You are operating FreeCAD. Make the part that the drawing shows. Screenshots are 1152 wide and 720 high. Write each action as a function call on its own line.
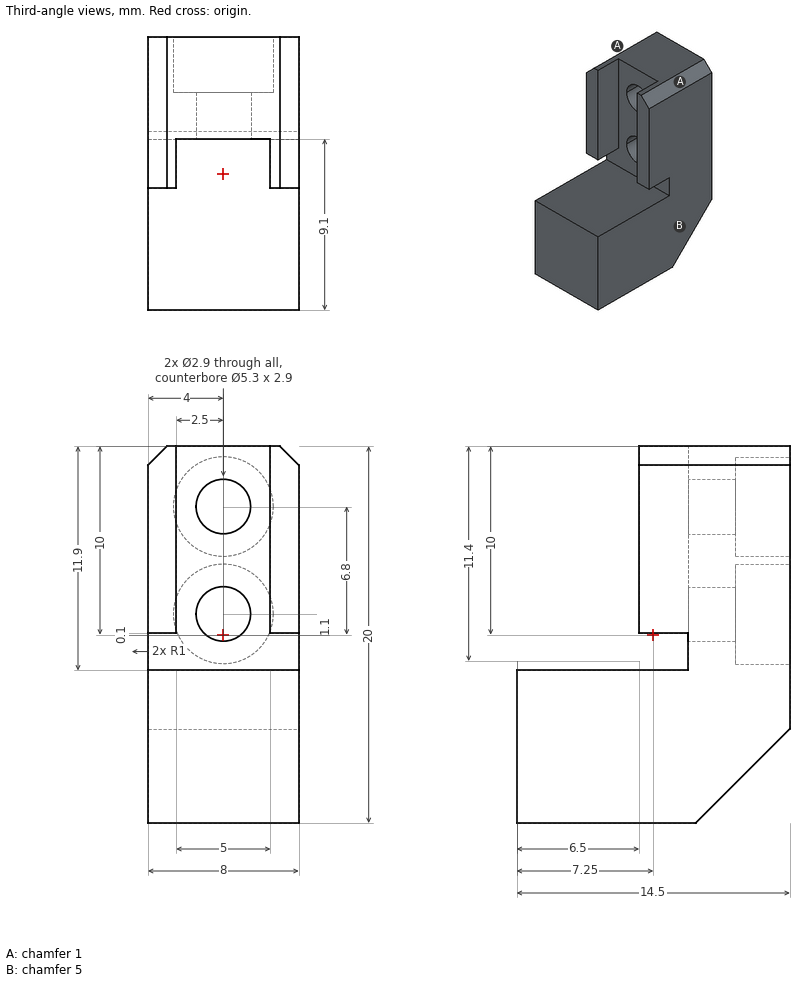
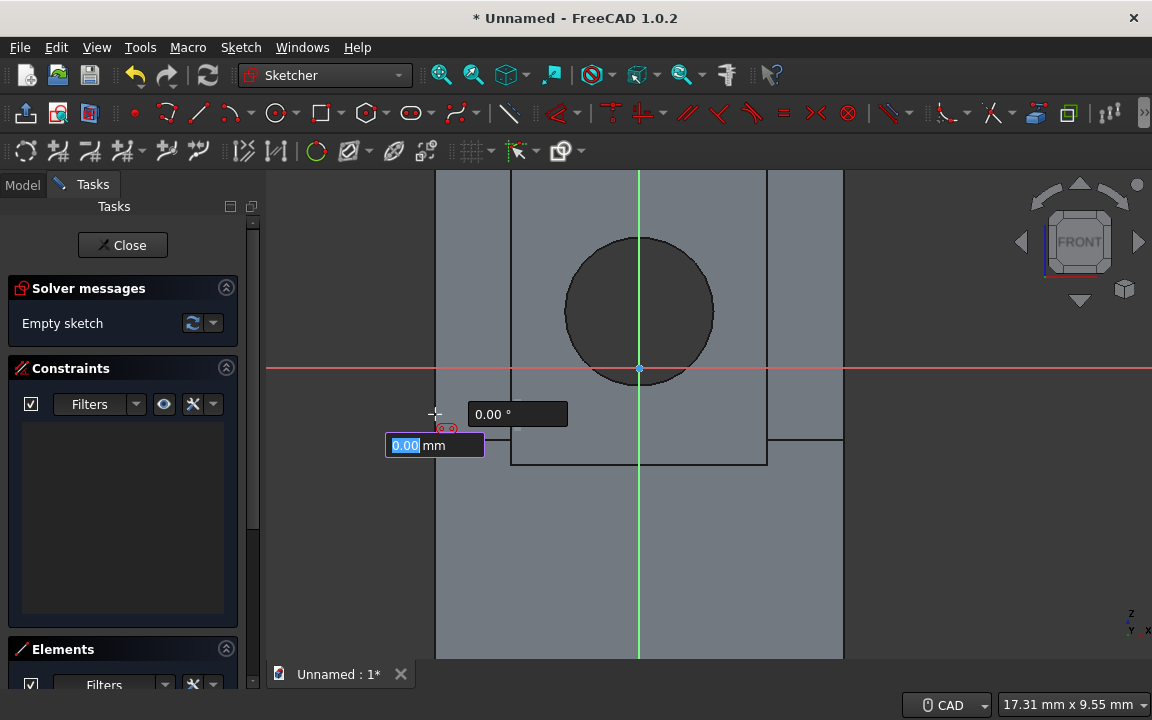
click(844, 414)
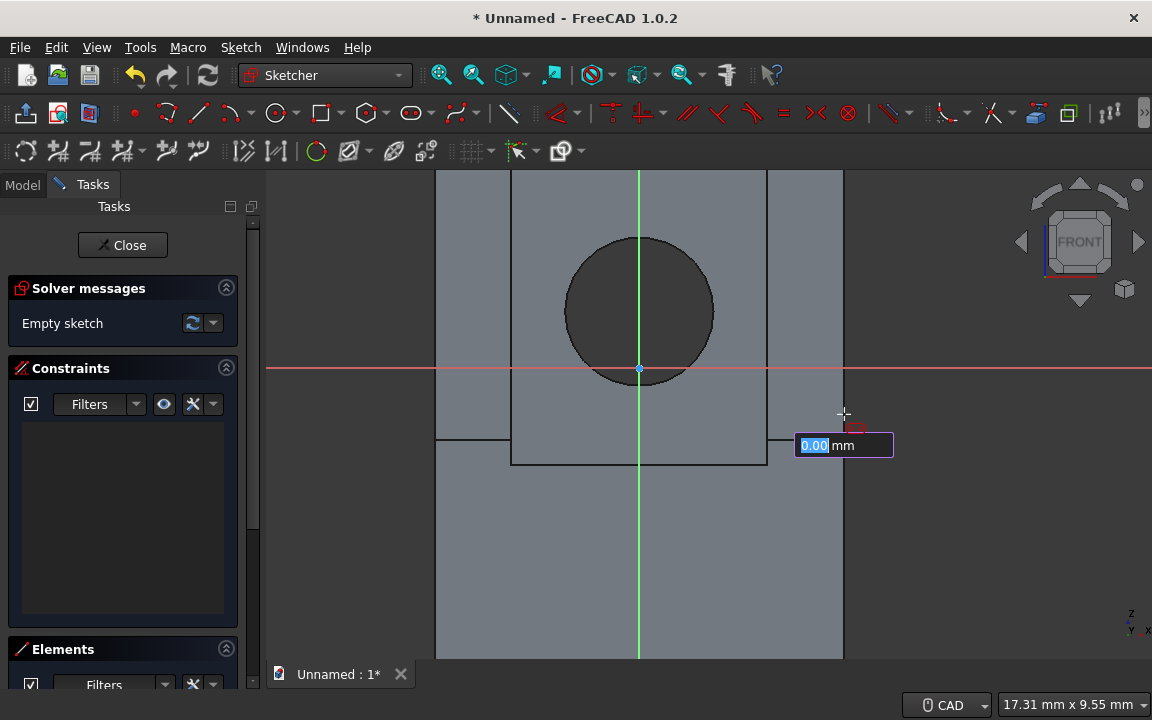
click(578, 465)
key(Escape)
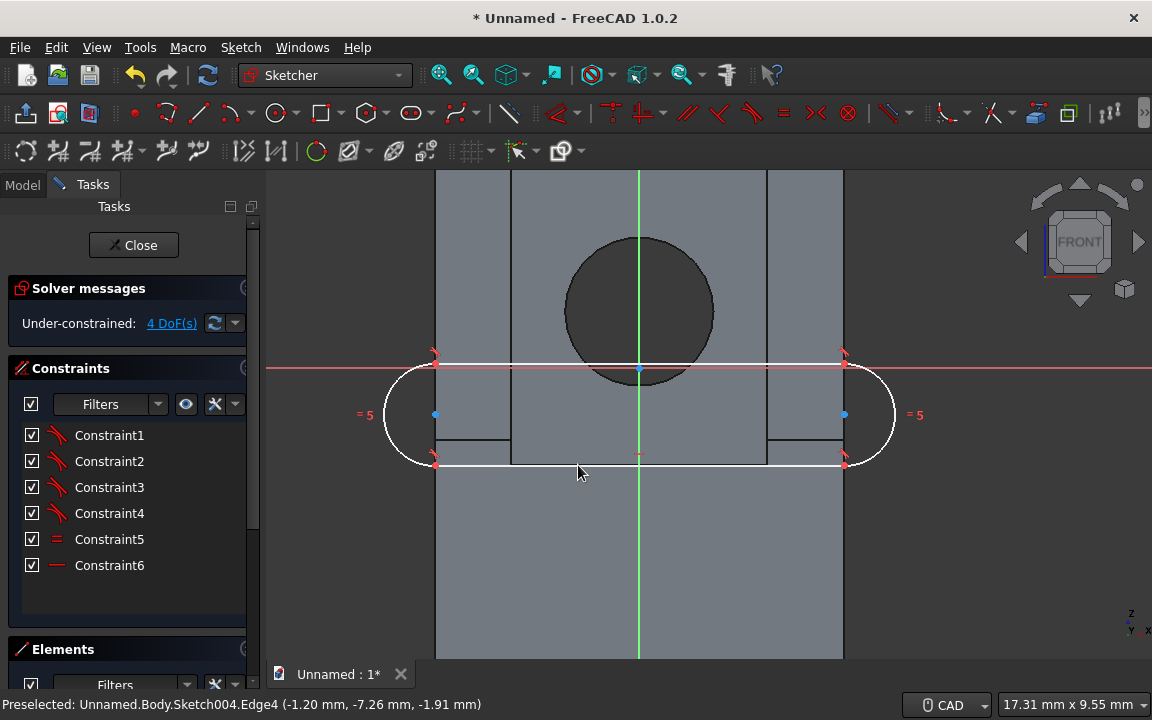
key(d)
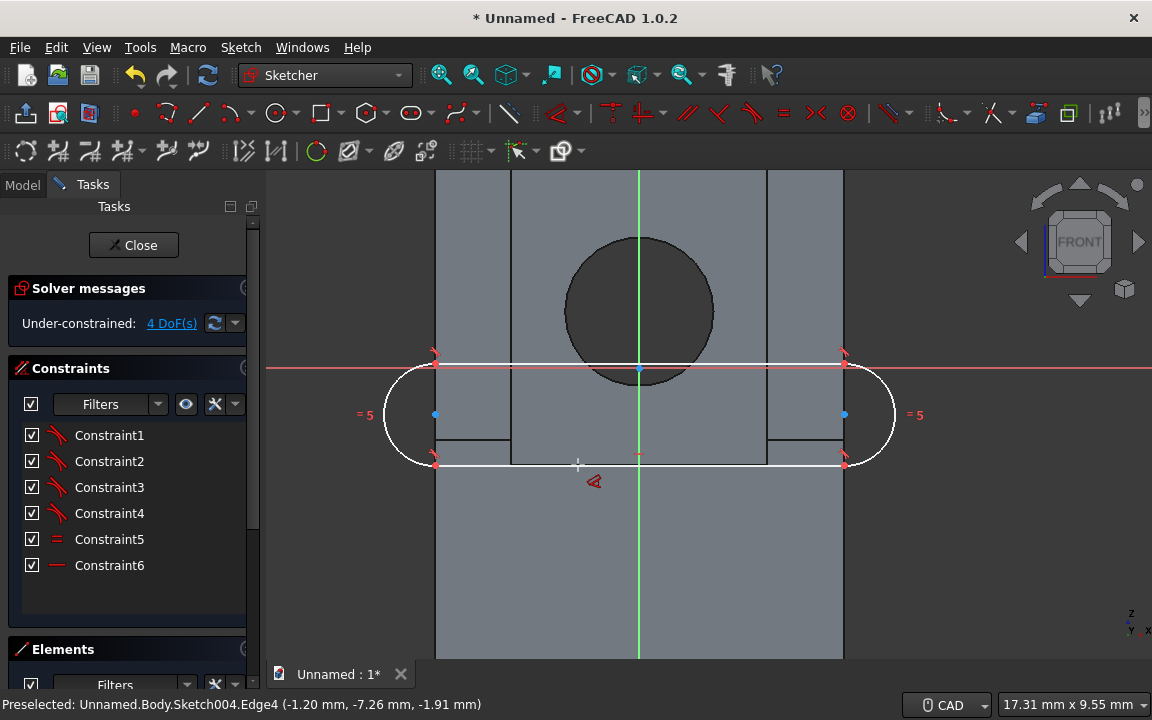
click(394, 385)
click(400, 340)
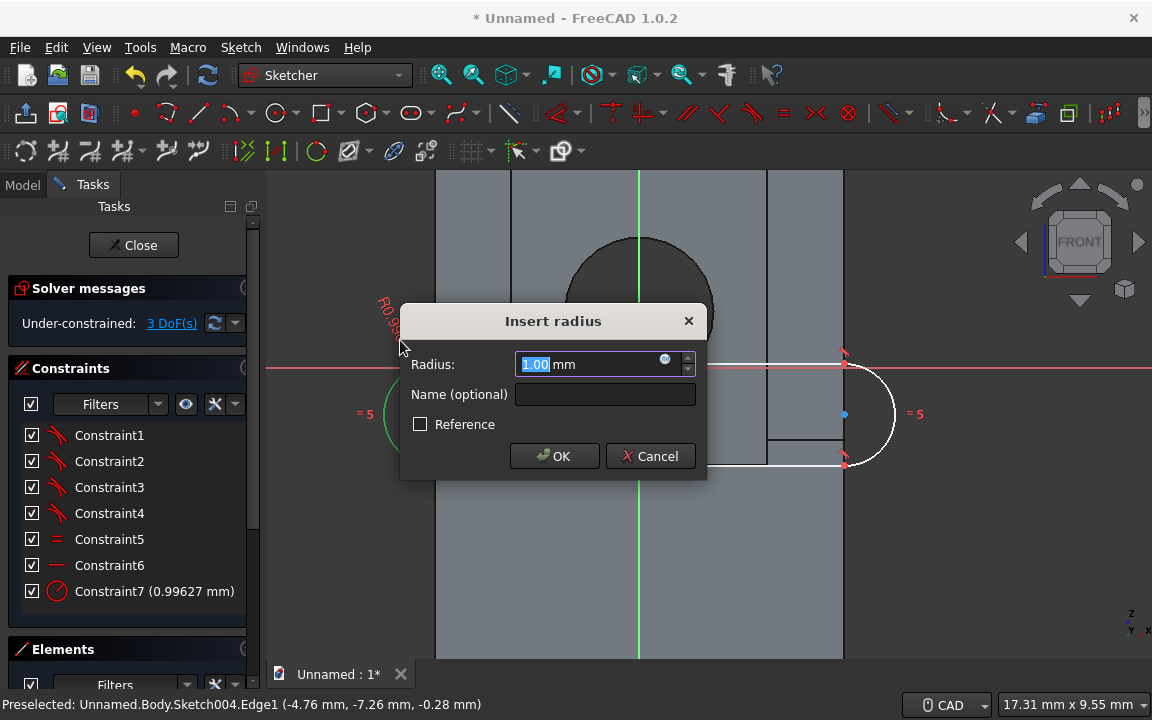
text(1)
key(Return)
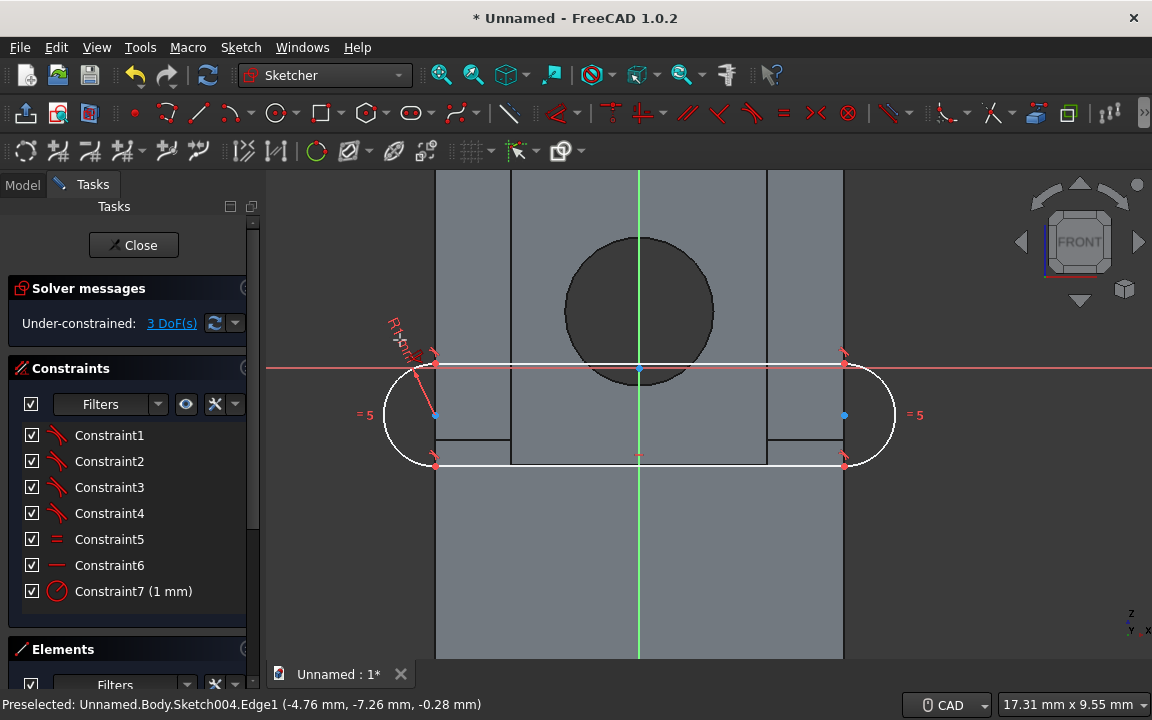
scroll(558, 364, up, 7)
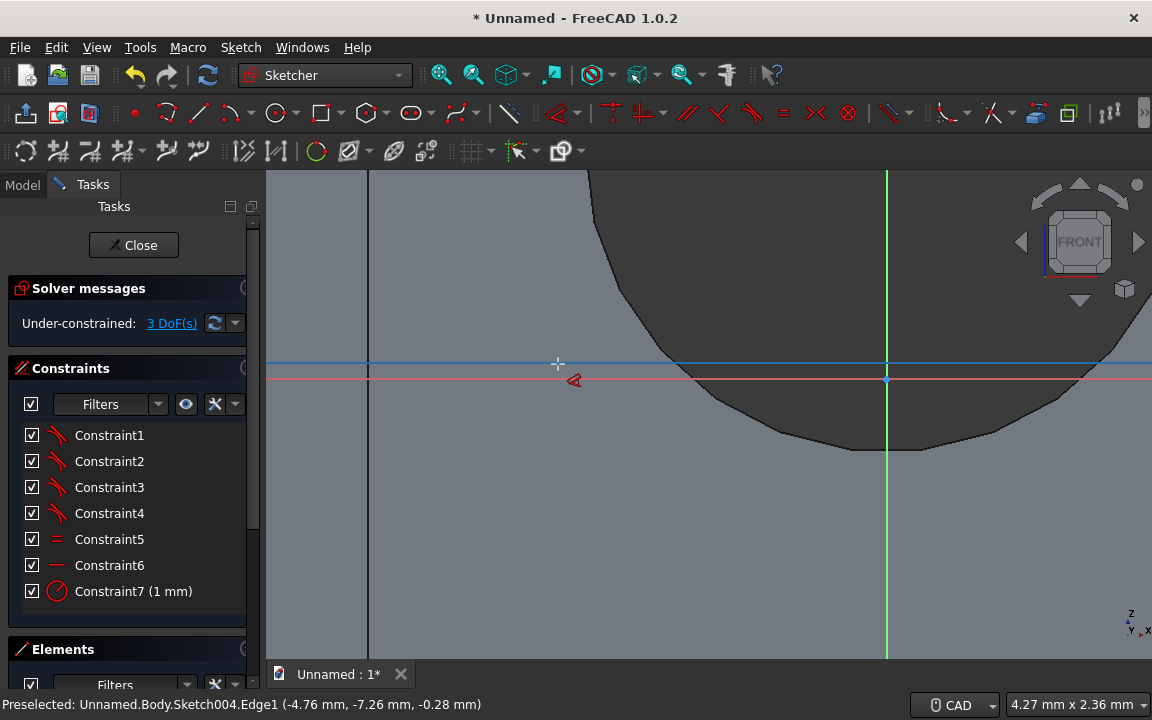
click(556, 363)
click(640, 329)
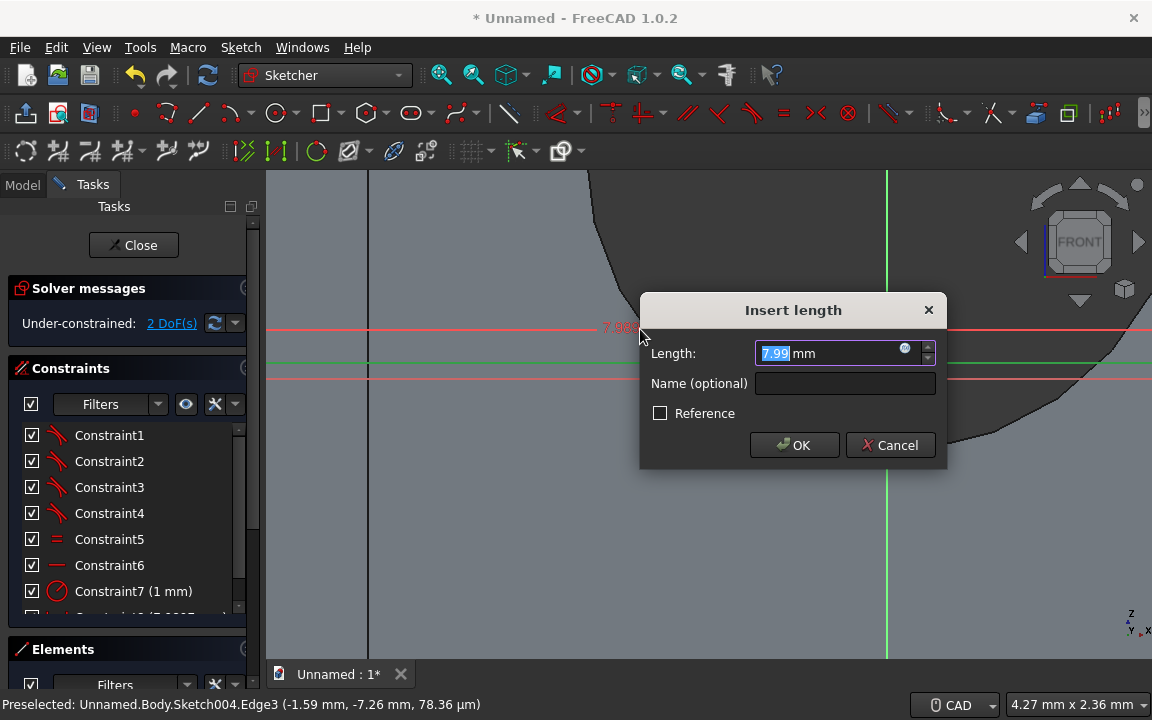
text(8)
key(Return)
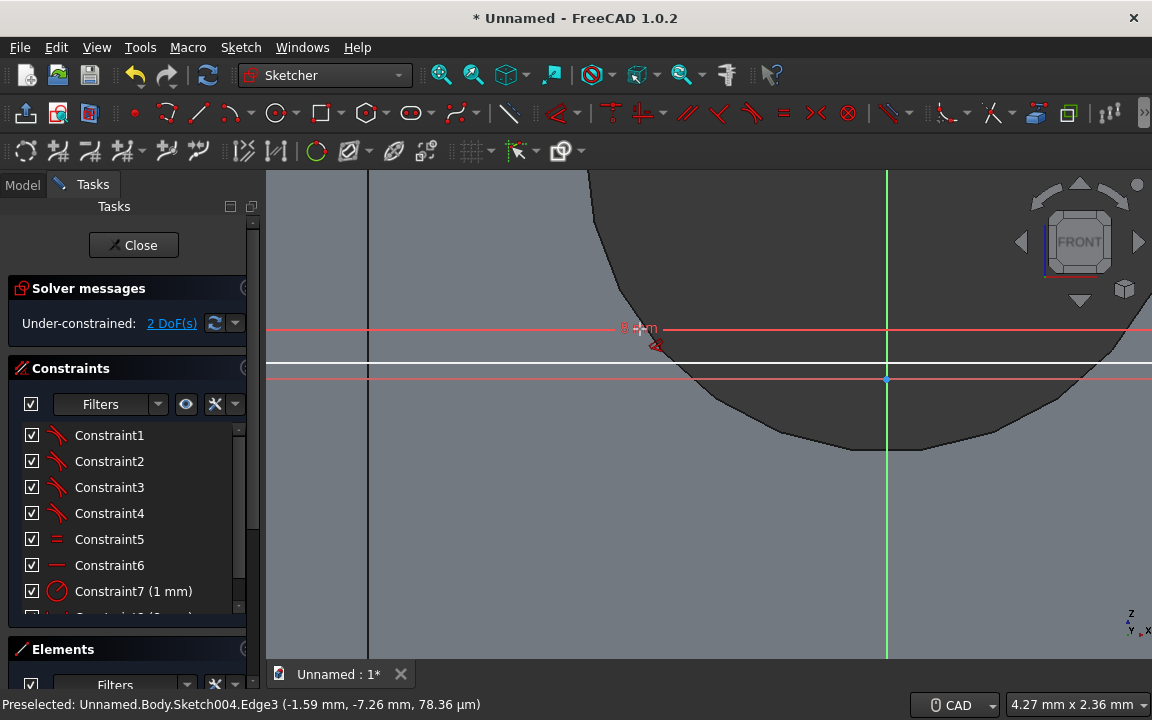
scroll(560, 365, down, 7)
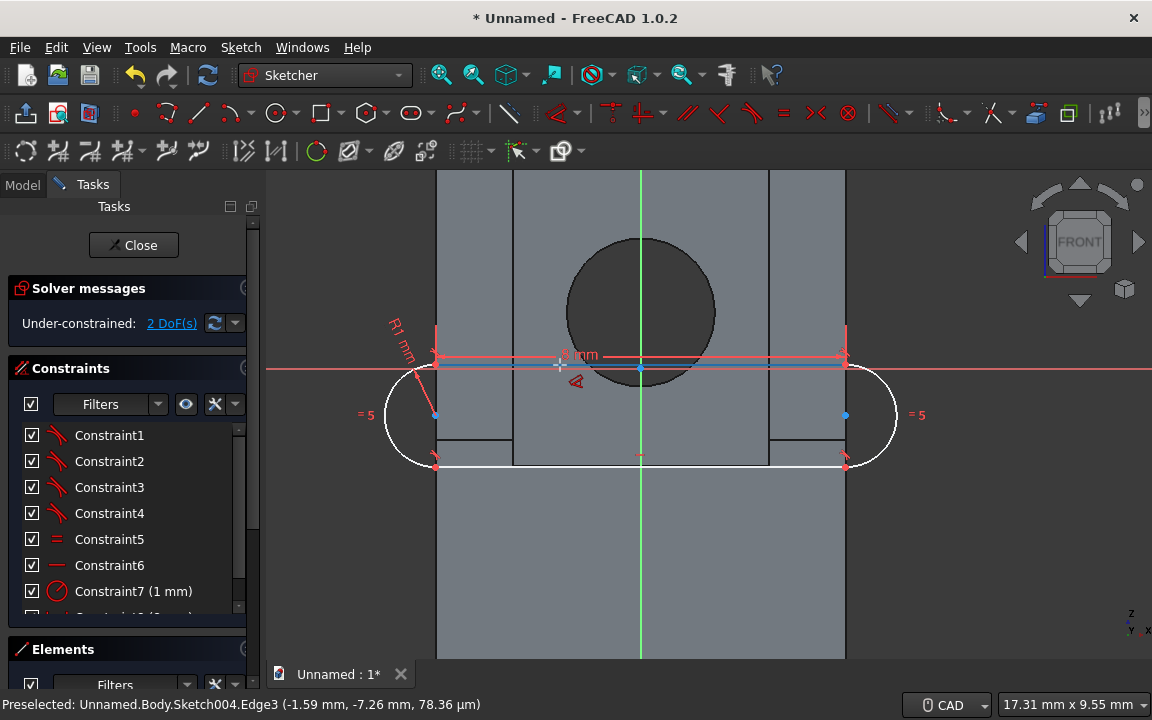
click(436, 365)
click(538, 331)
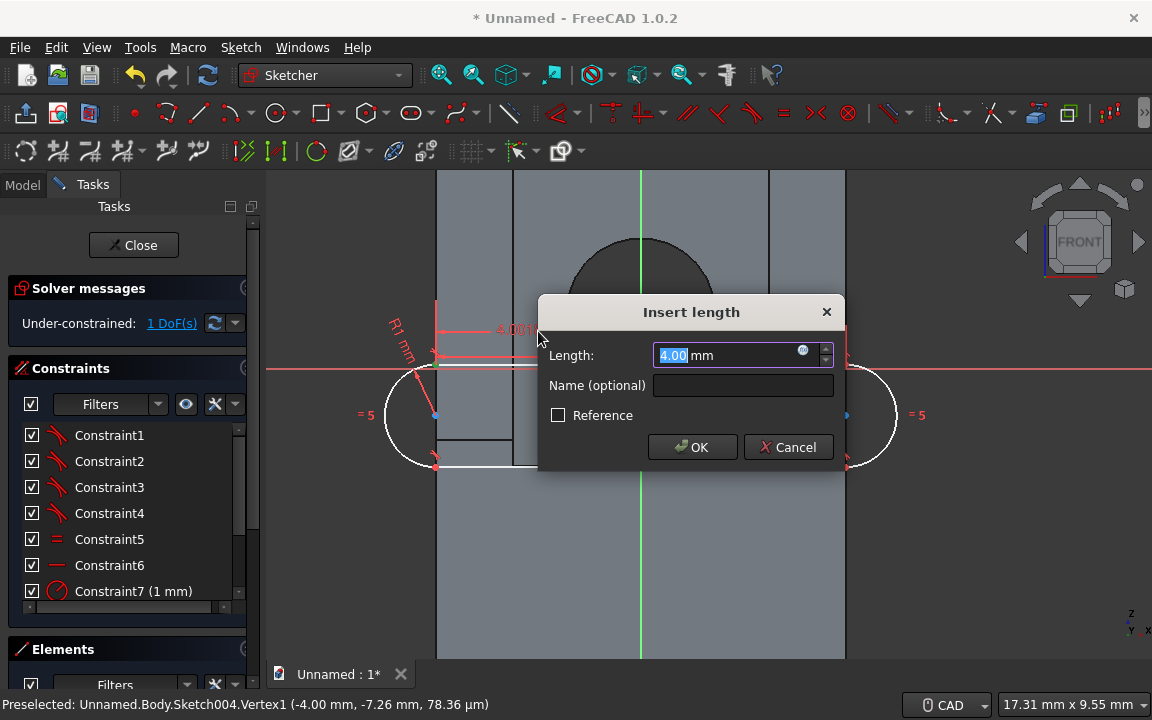
text(4)
key(Return)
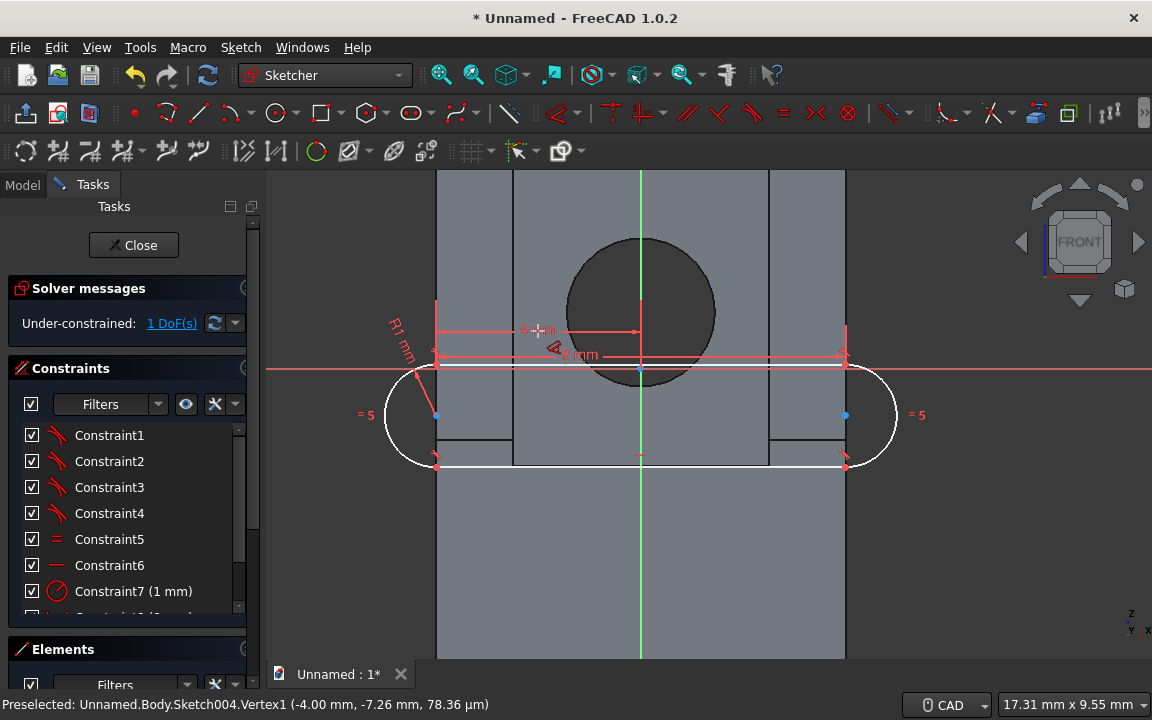
scroll(436, 365, up, 11)